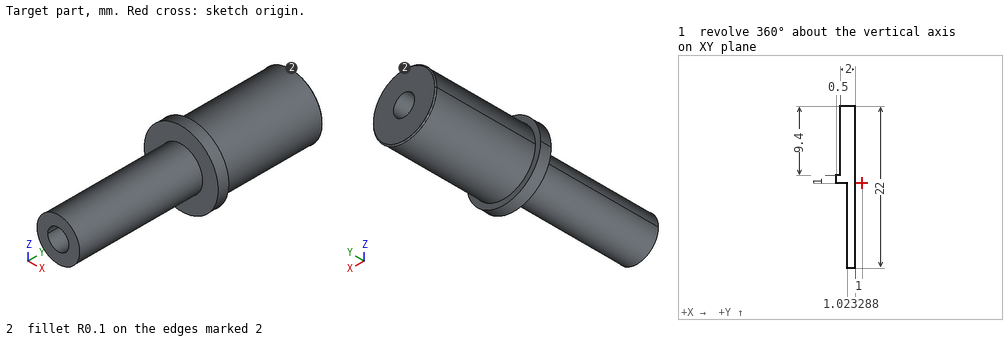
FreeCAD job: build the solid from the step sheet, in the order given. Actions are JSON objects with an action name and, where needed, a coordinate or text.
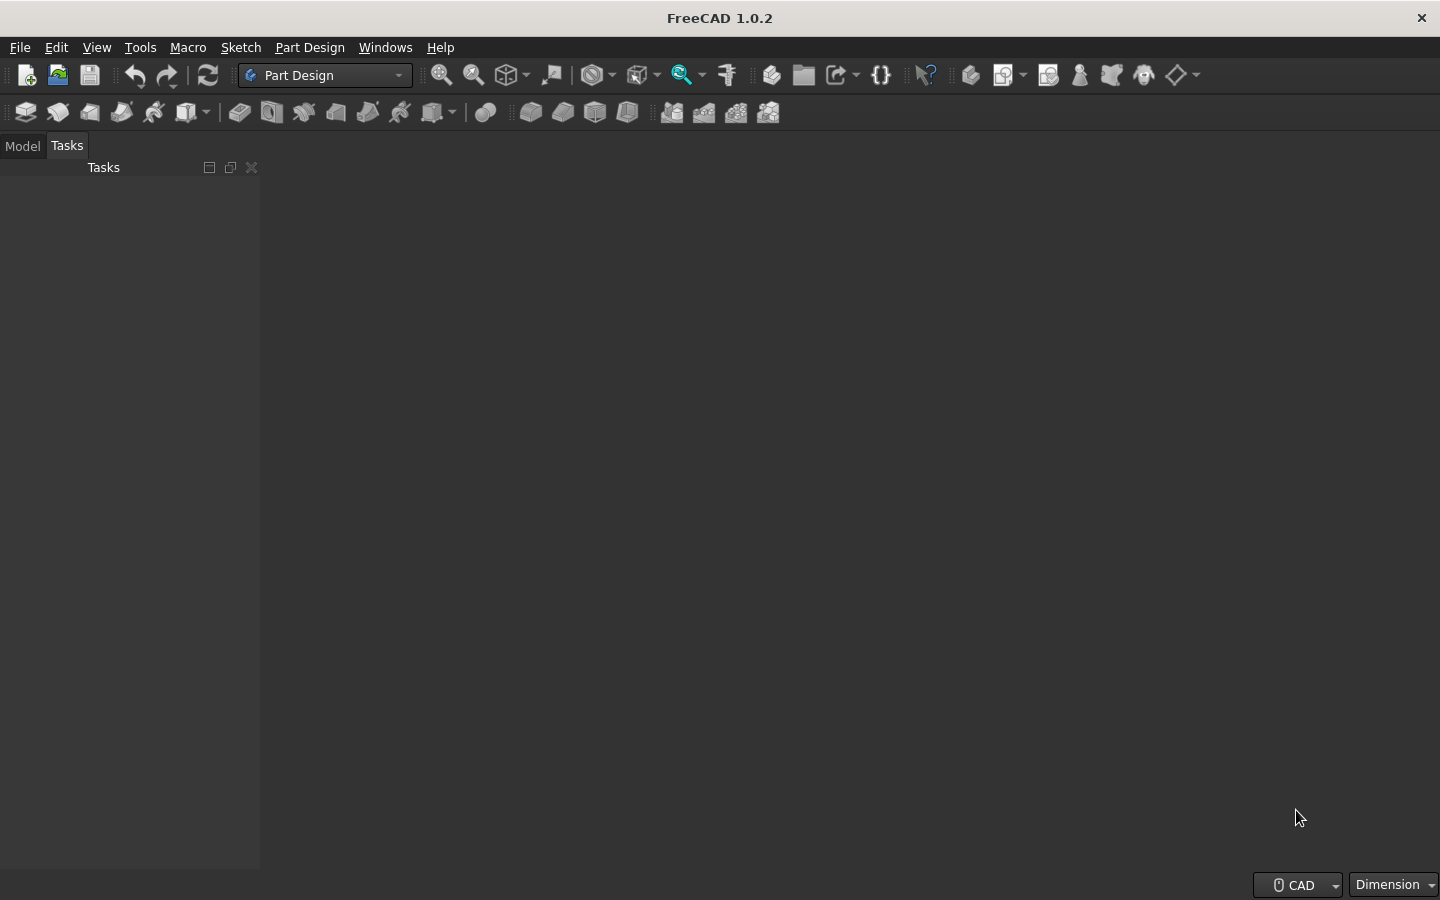
{"action": "key", "text": "ctrl+n"}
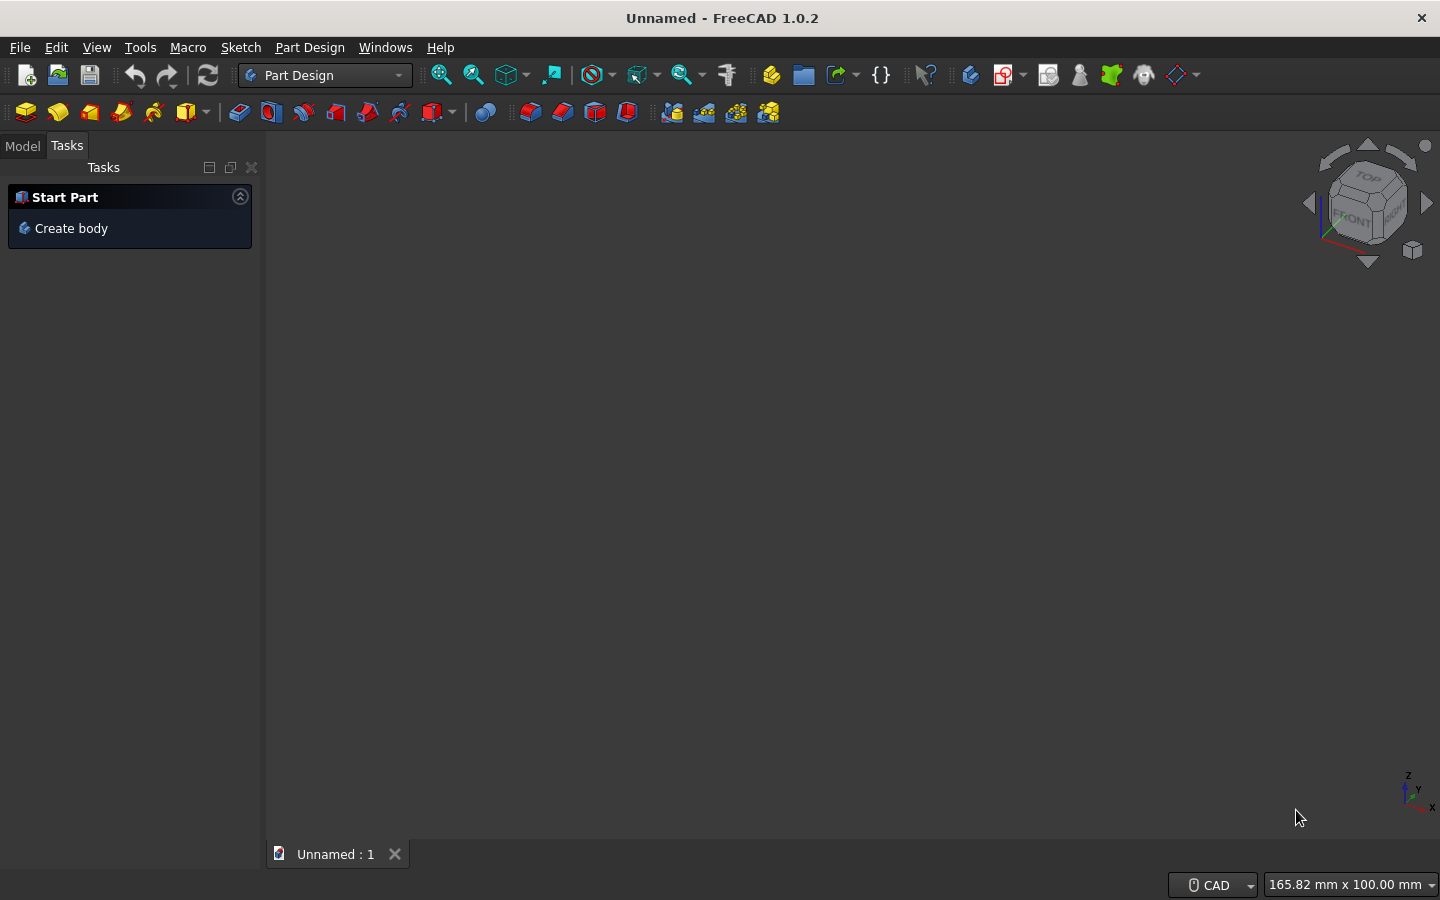
{"action": "left_click", "coordinate": [1004, 76]}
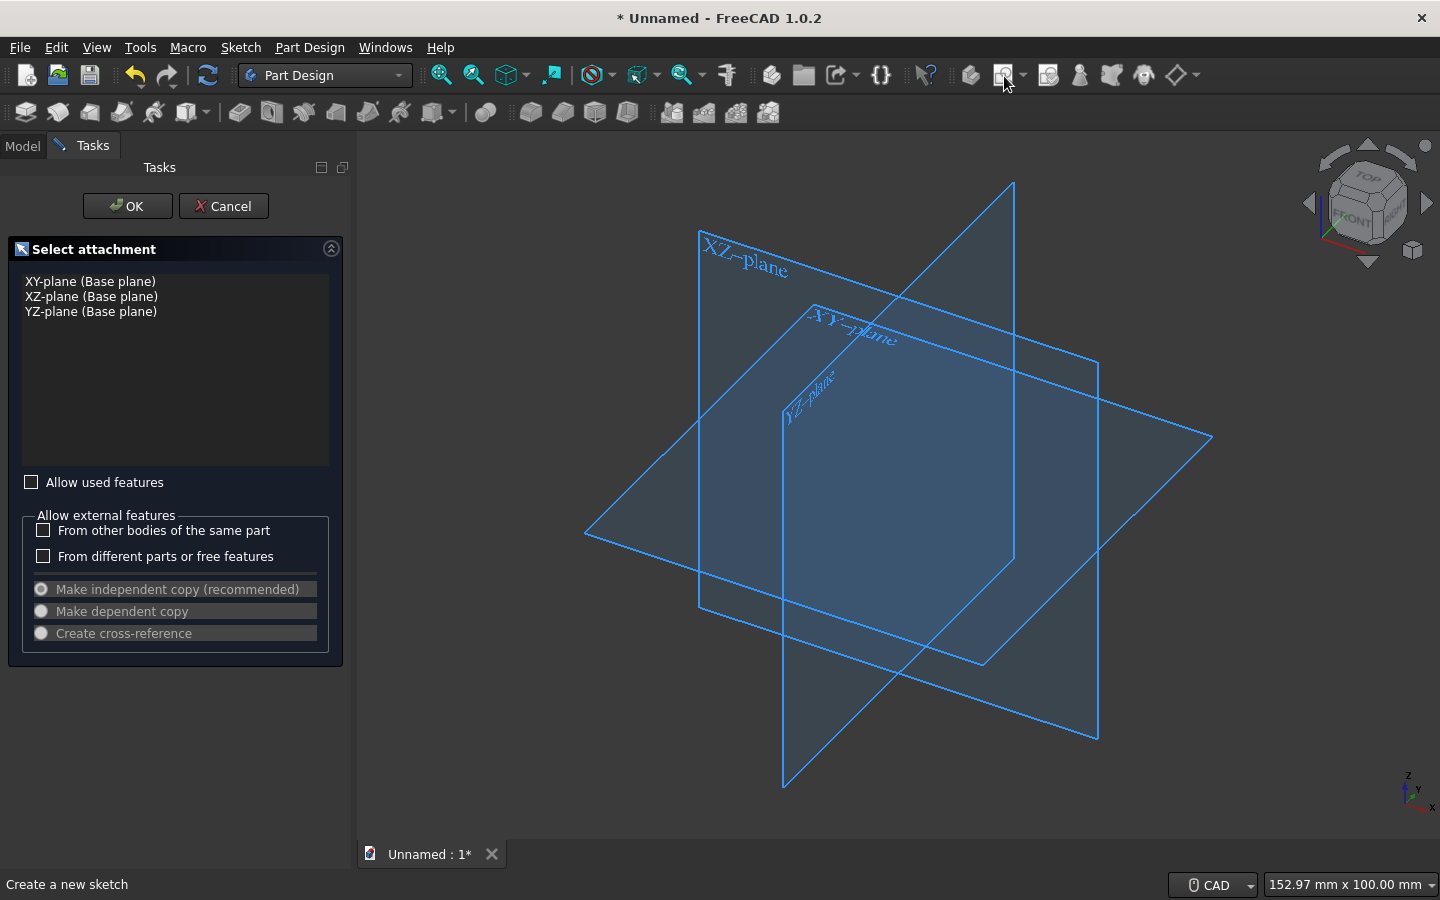
{"action": "left_click", "coordinate": [82, 282]}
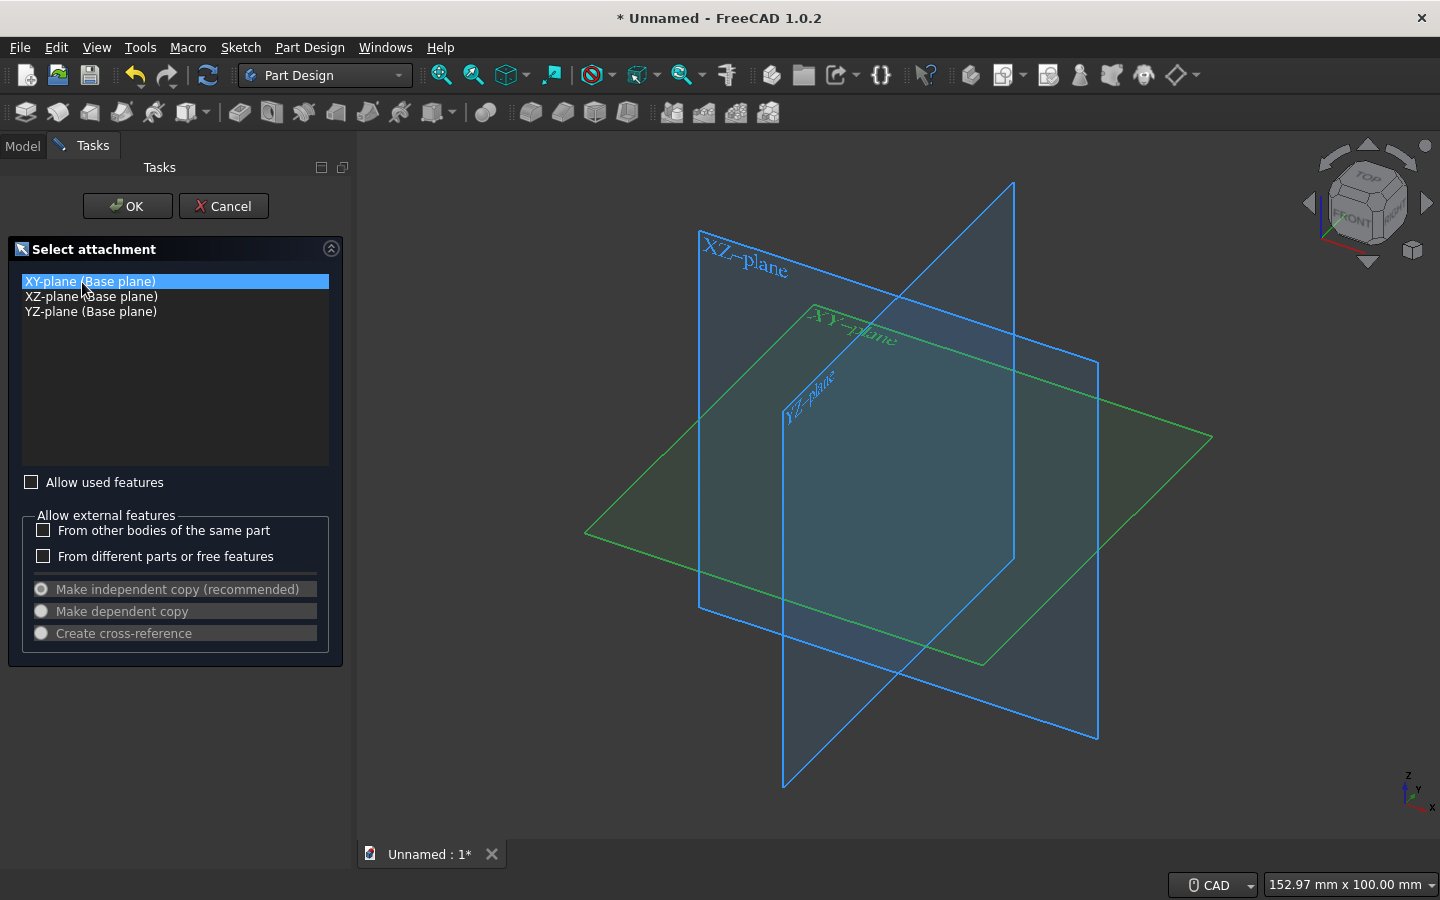
{"action": "left_click", "coordinate": [128, 206]}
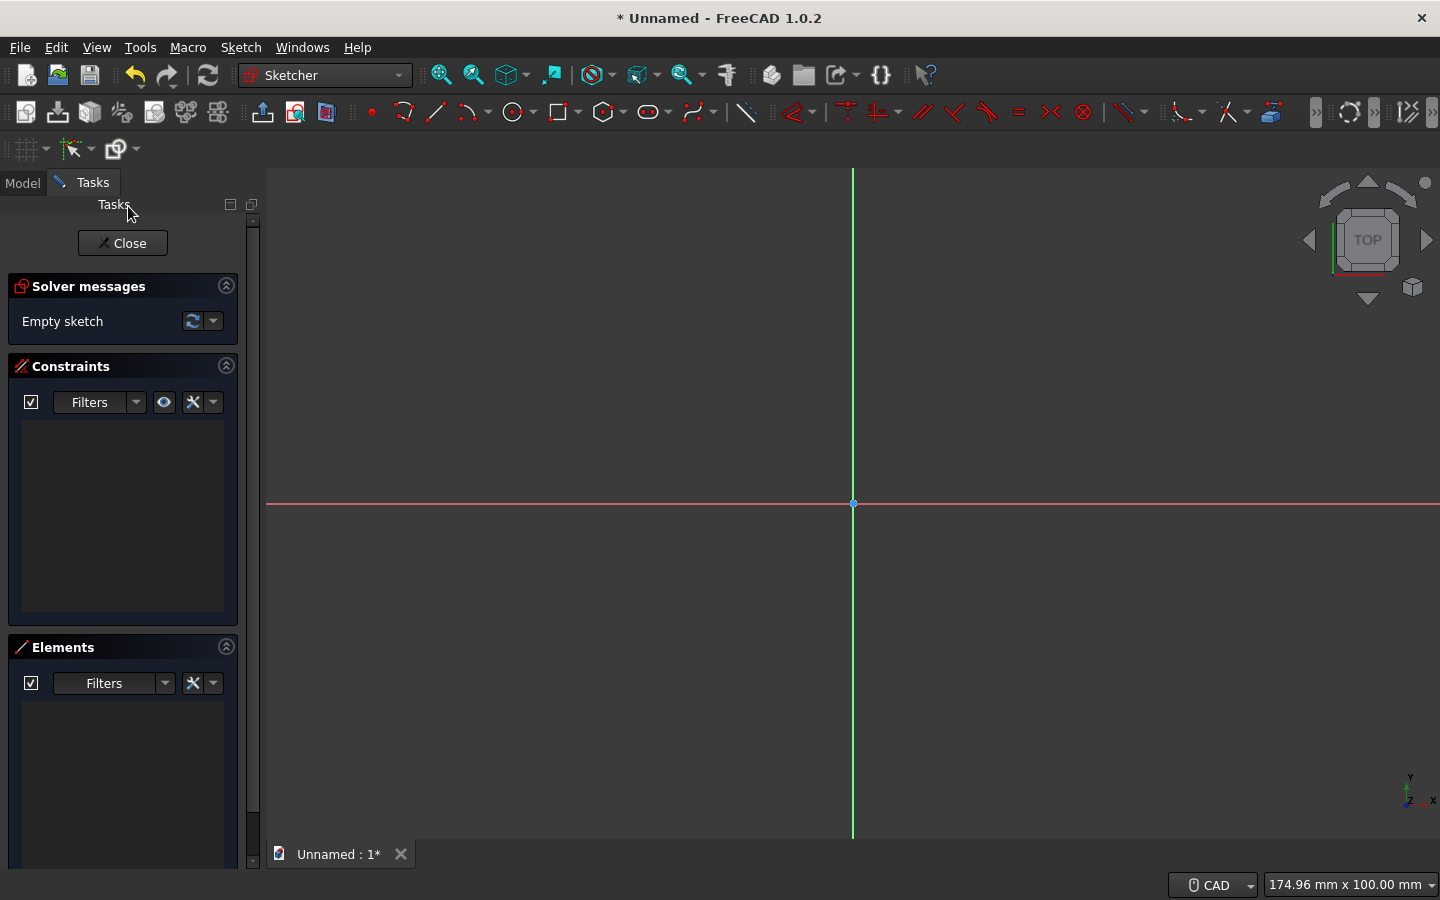
{"action": "scroll", "coordinate": [874, 510], "scroll_direction": "up", "scroll_amount": 5}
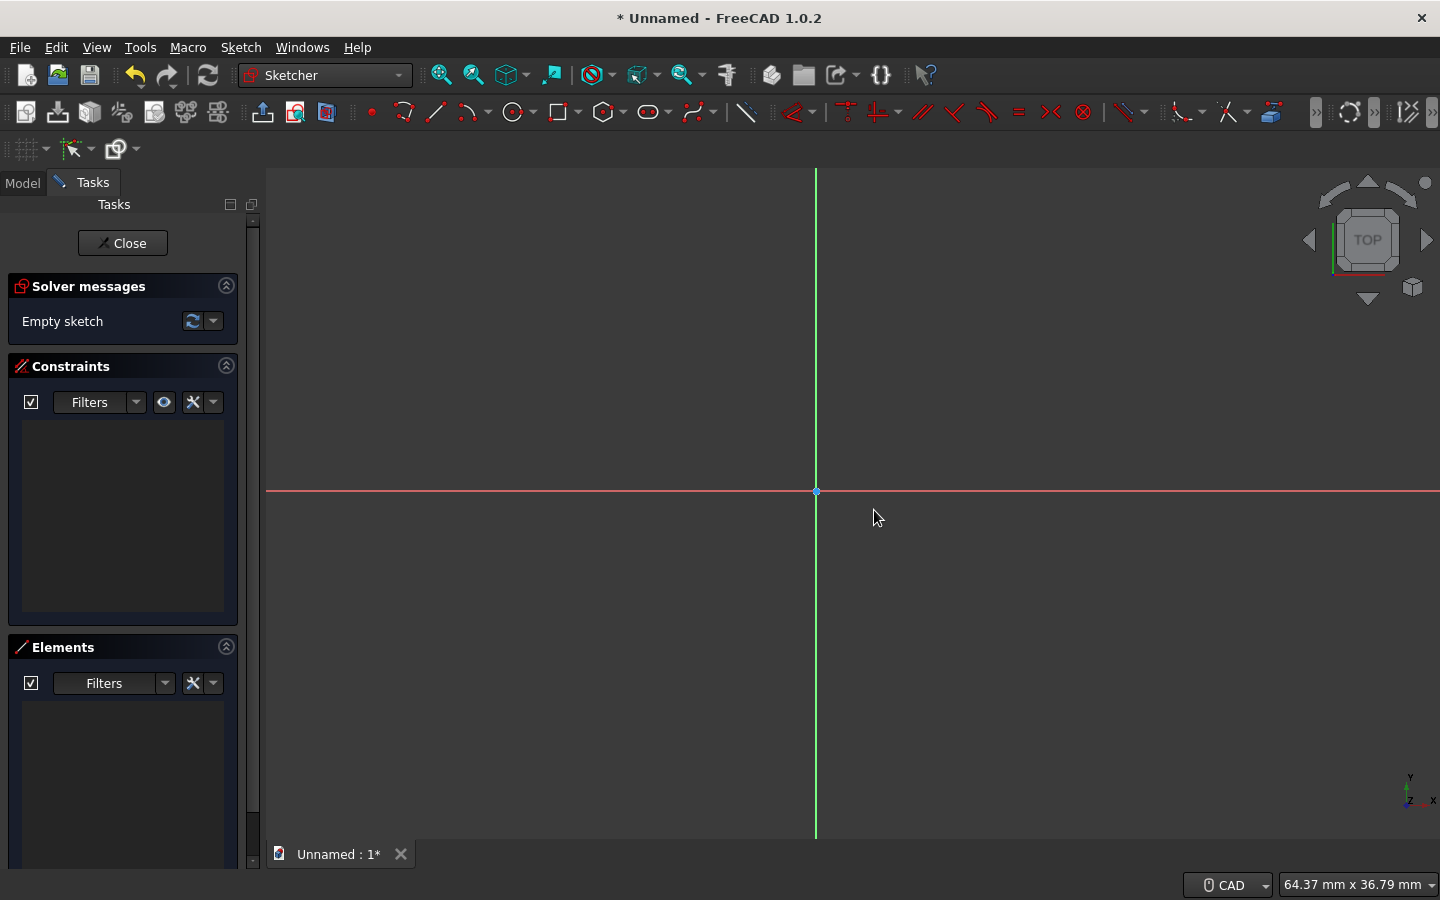
{"action": "left_click", "coordinate": [404, 112]}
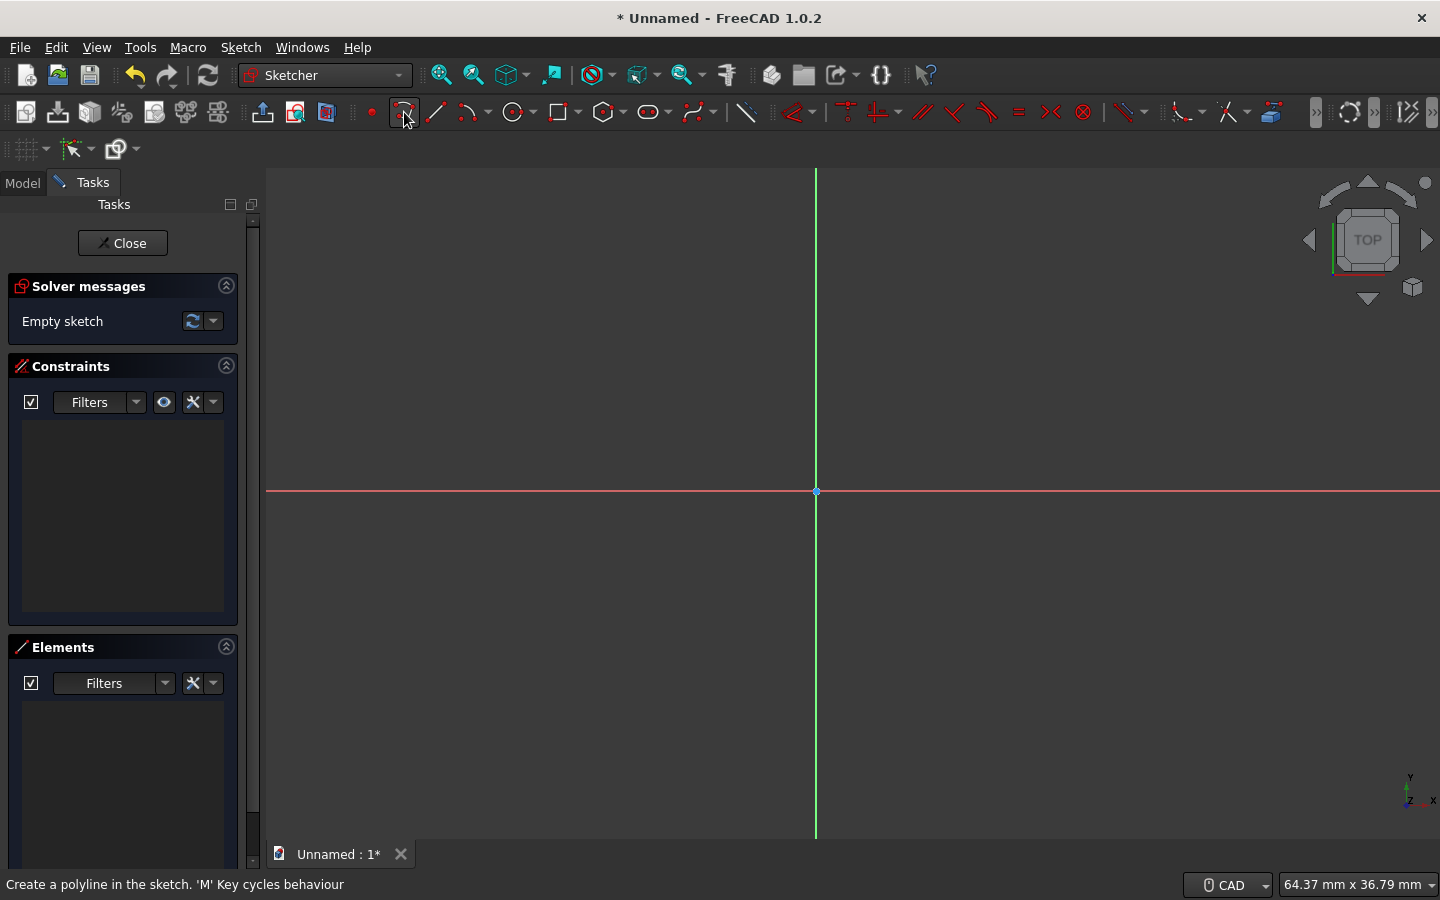
{"action": "left_click", "coordinate": [779, 491]}
{"action": "left_click", "coordinate": [779, 703]}
{"action": "left_click", "coordinate": [798, 703]}
{"action": "left_click", "coordinate": [798, 302]}
{"action": "left_click", "coordinate": [761, 302]}
{"action": "left_click", "coordinate": [761, 473]}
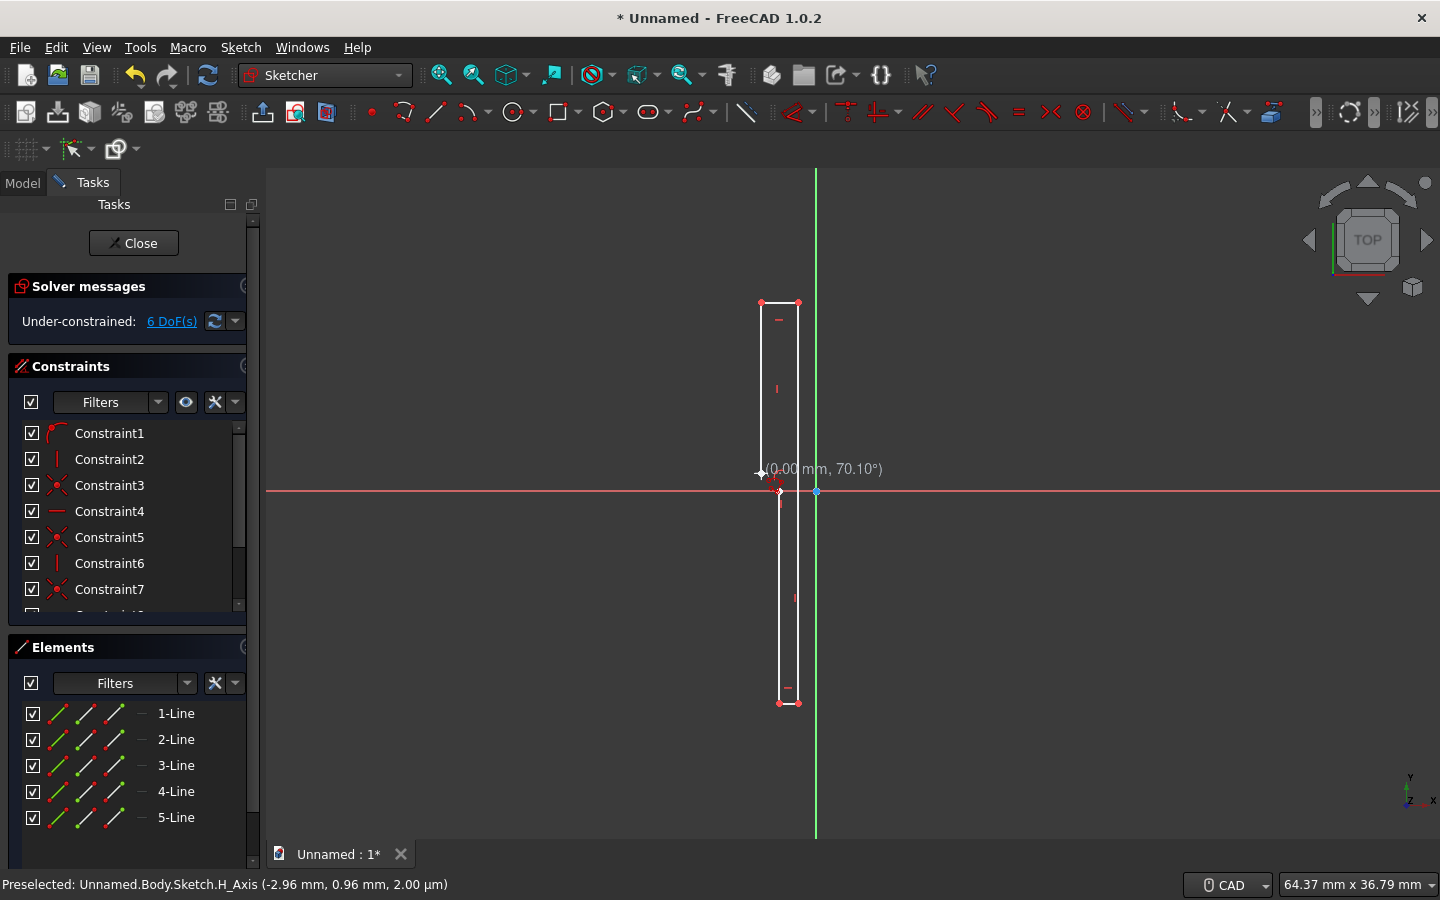
{"action": "scroll", "coordinate": [752, 473], "scroll_direction": "up", "scroll_amount": 3}